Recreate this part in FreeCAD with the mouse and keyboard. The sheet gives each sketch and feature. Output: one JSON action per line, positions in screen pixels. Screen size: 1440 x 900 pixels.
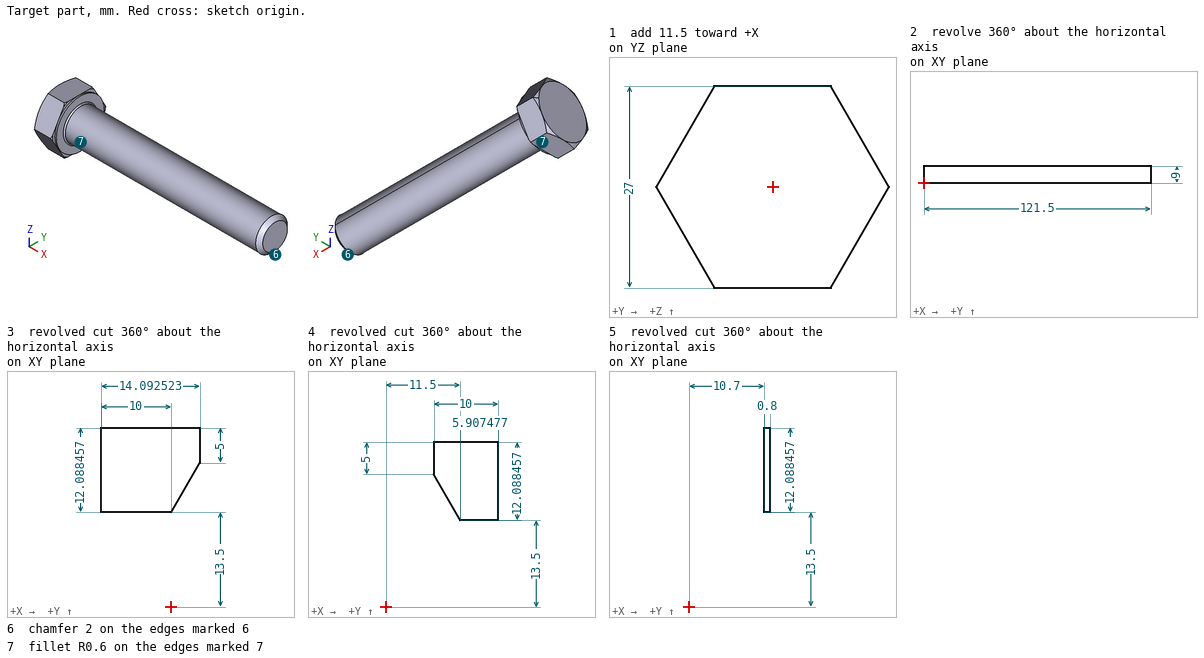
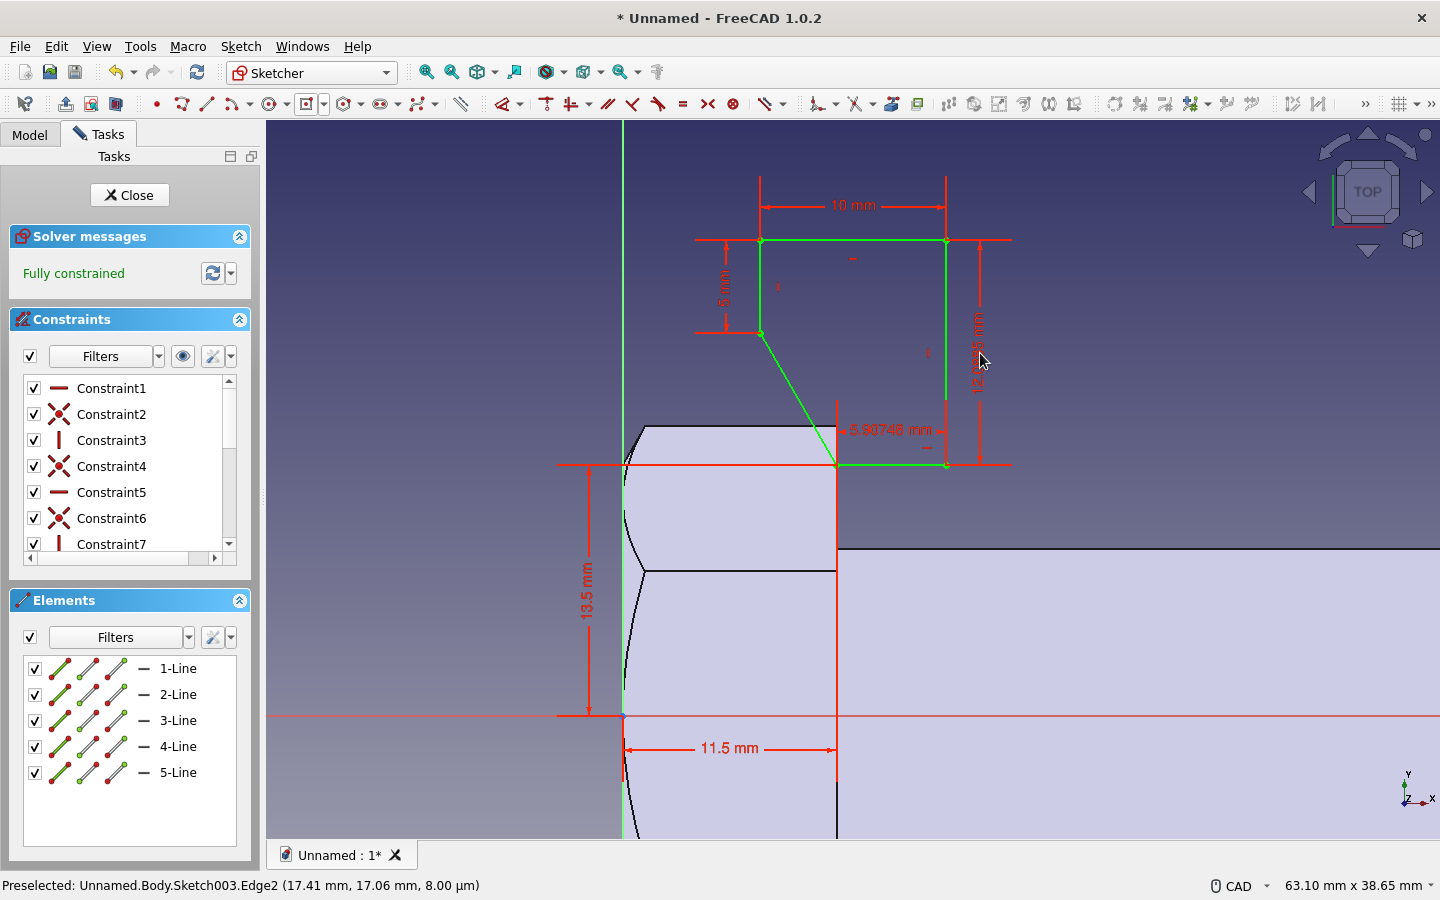
{"action": "left_click", "coordinate": [130, 195]}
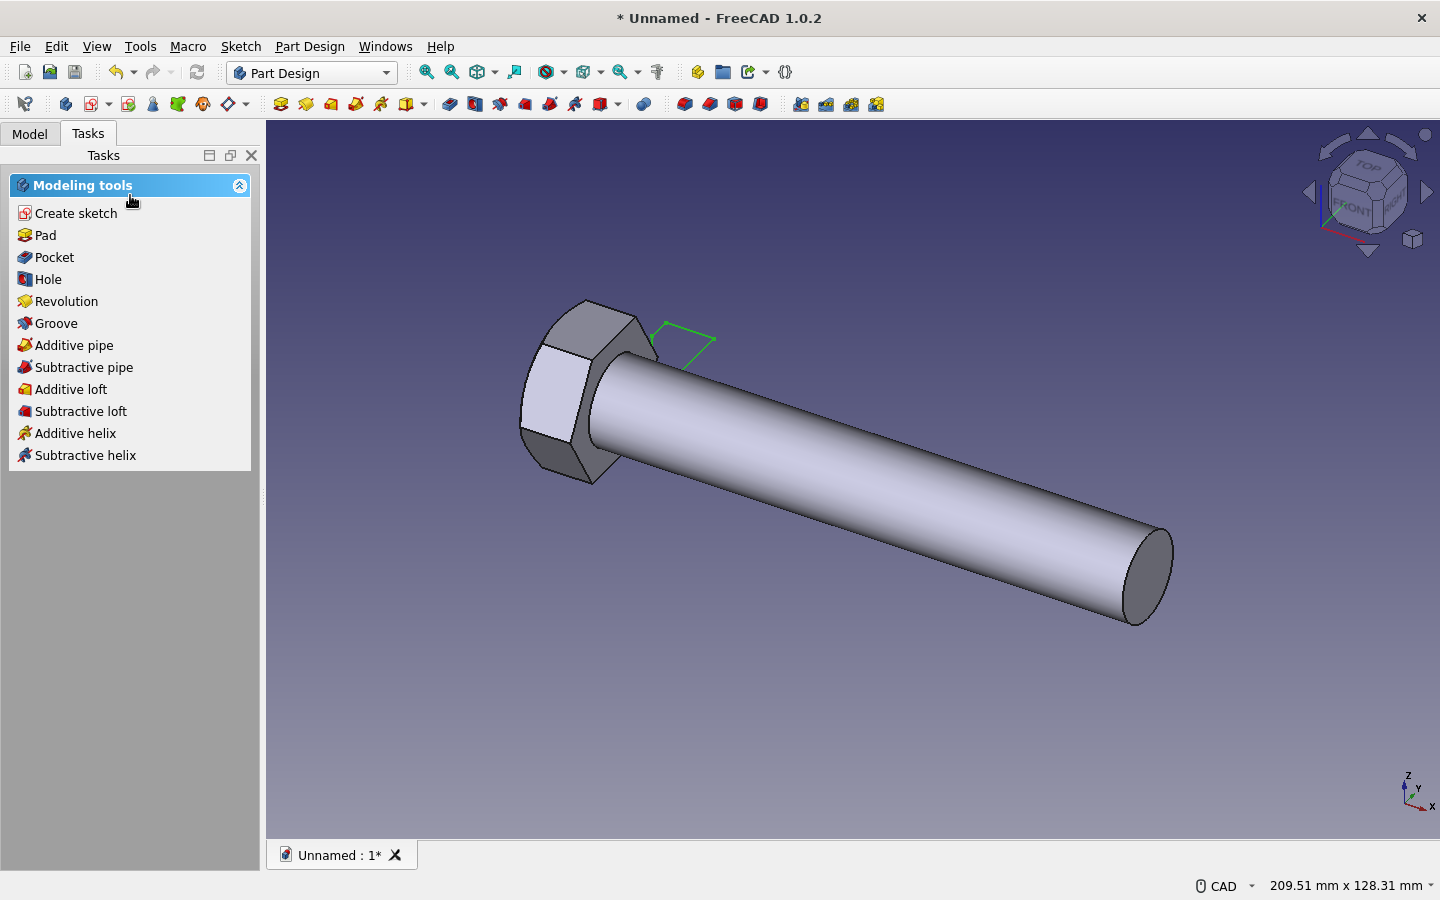
{"action": "left_click", "coordinate": [500, 104]}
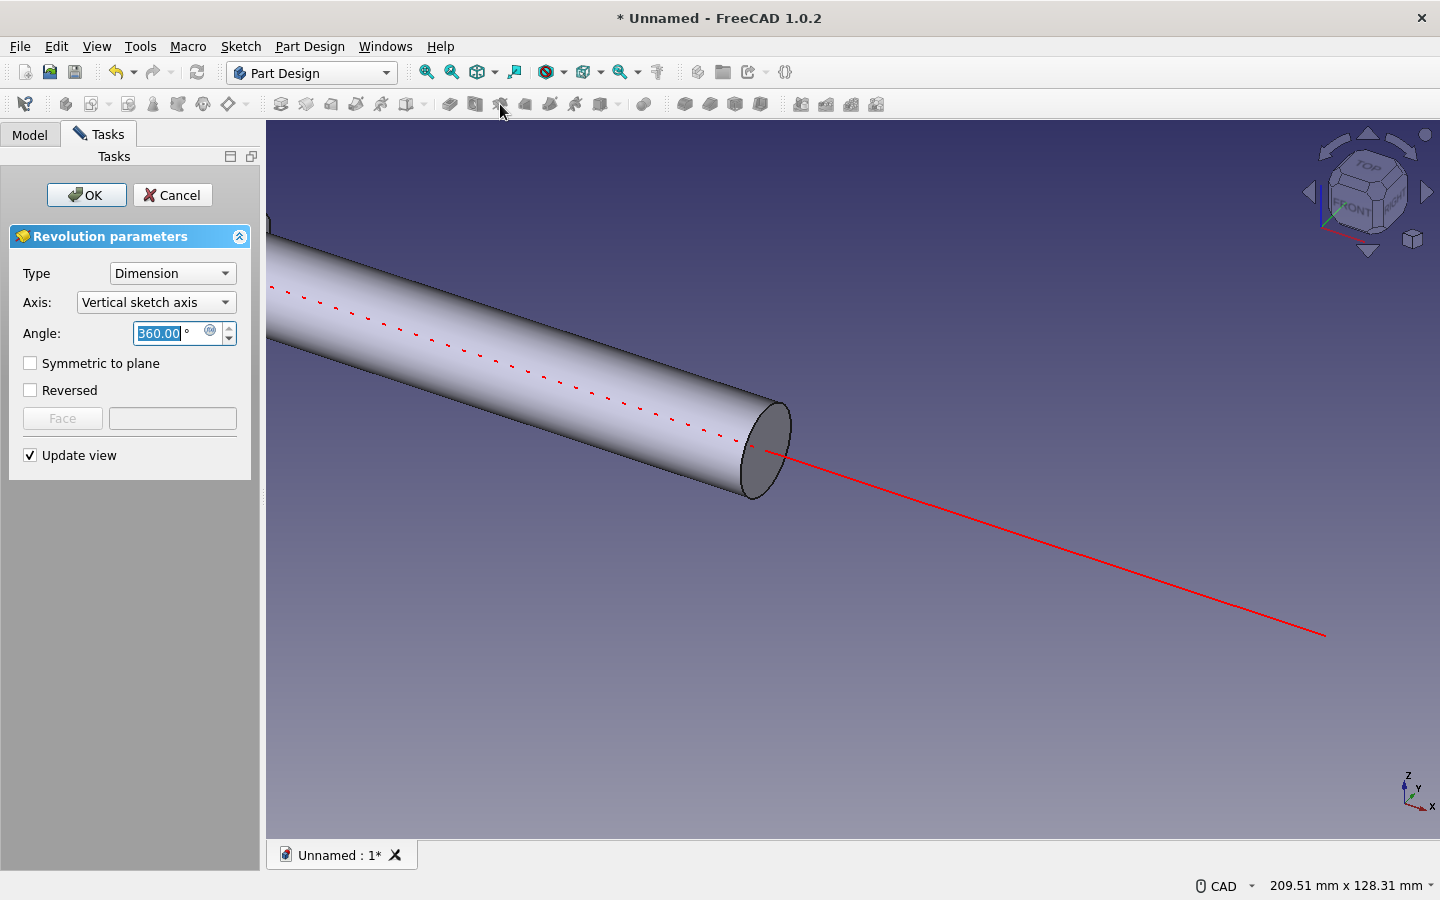
{"action": "left_click", "coordinate": [157, 302]}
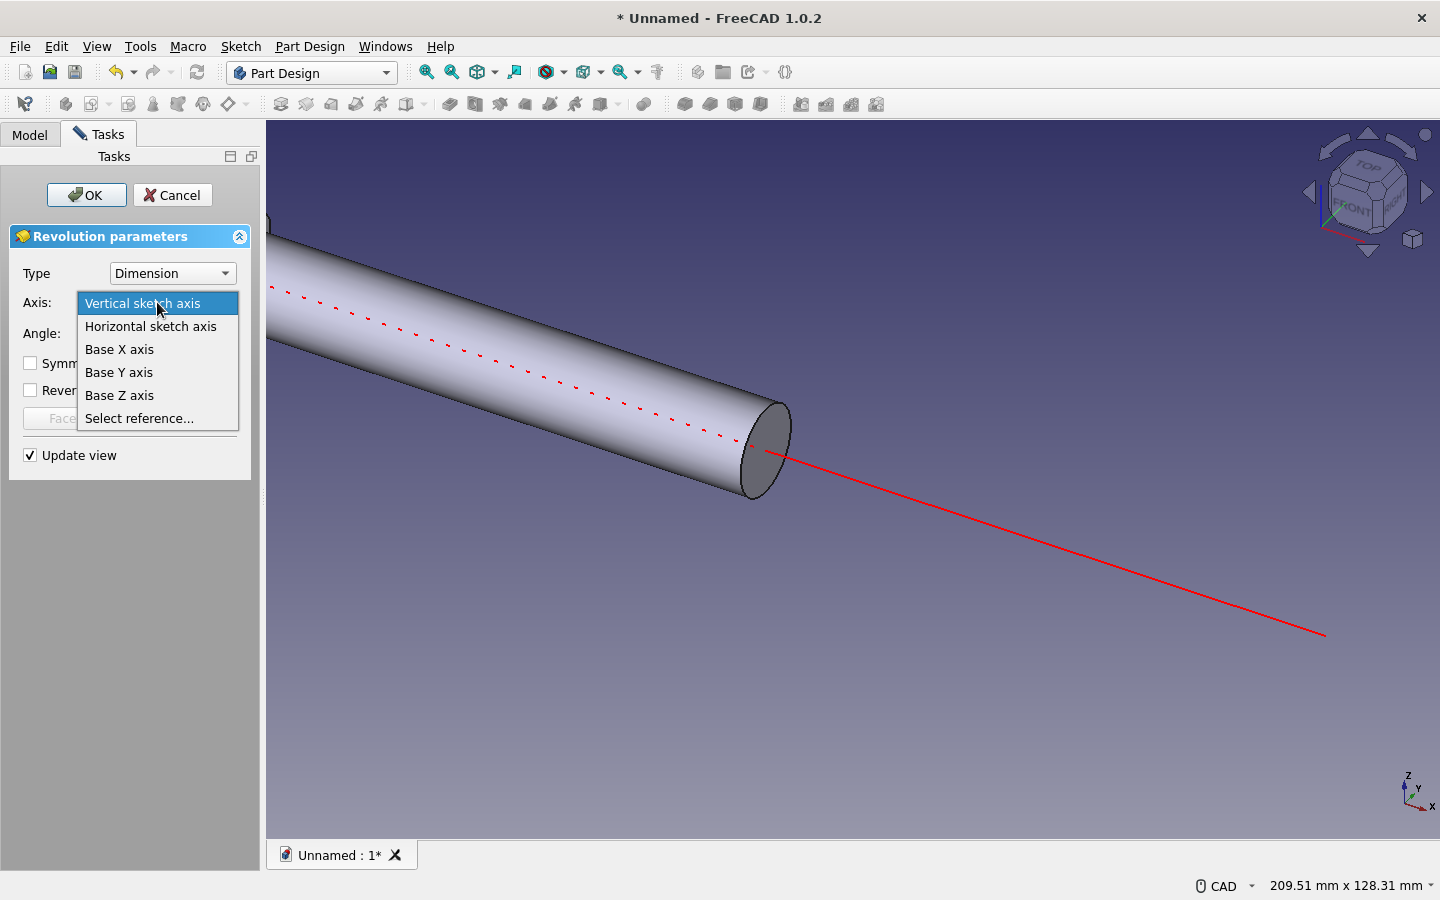
{"action": "left_click", "coordinate": [156, 326]}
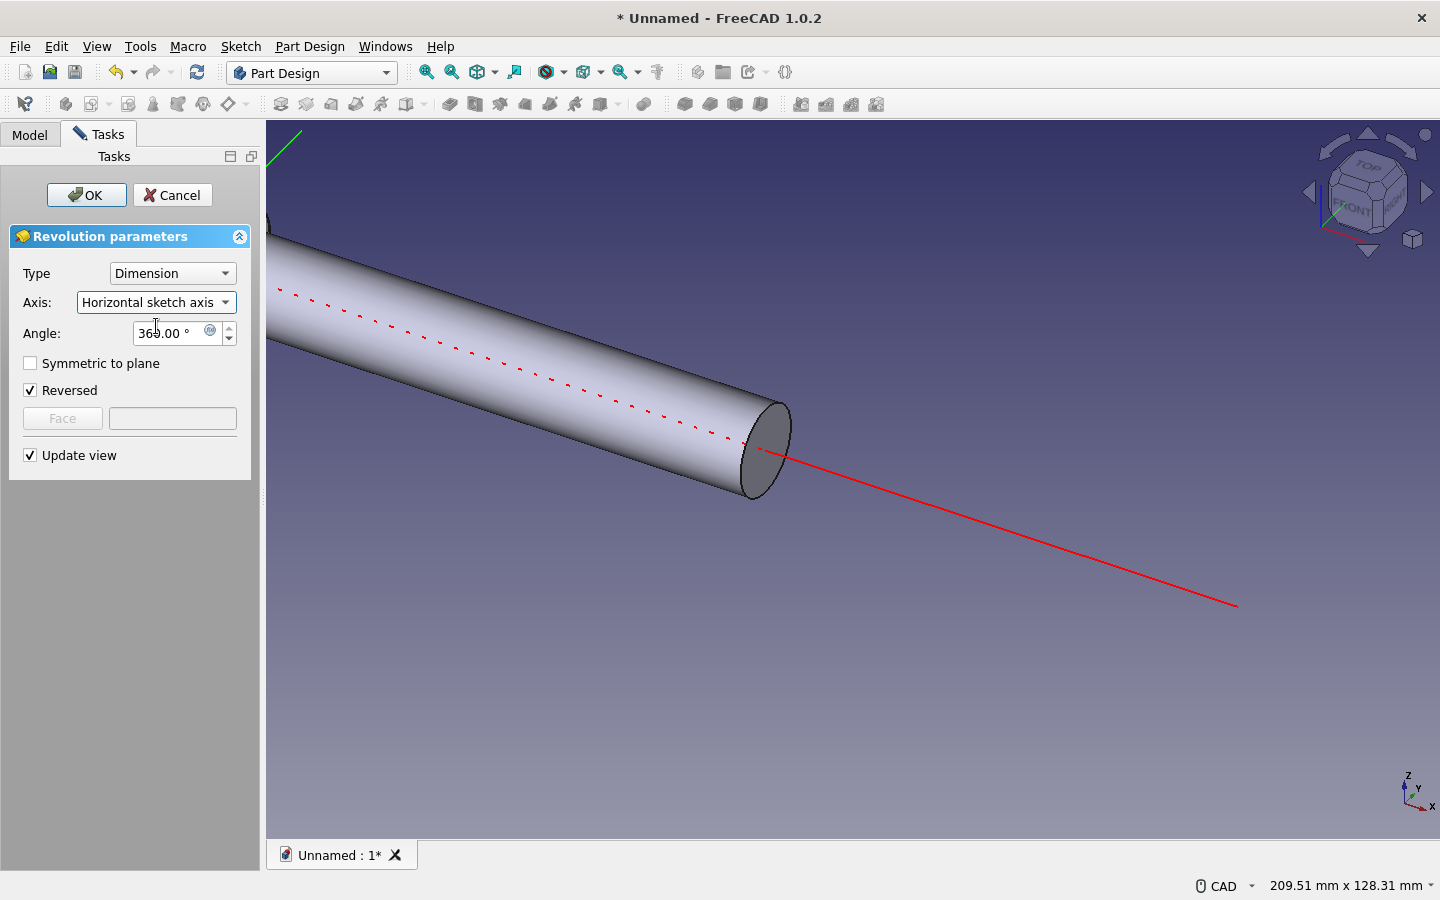
{"action": "left_click", "coordinate": [87, 195]}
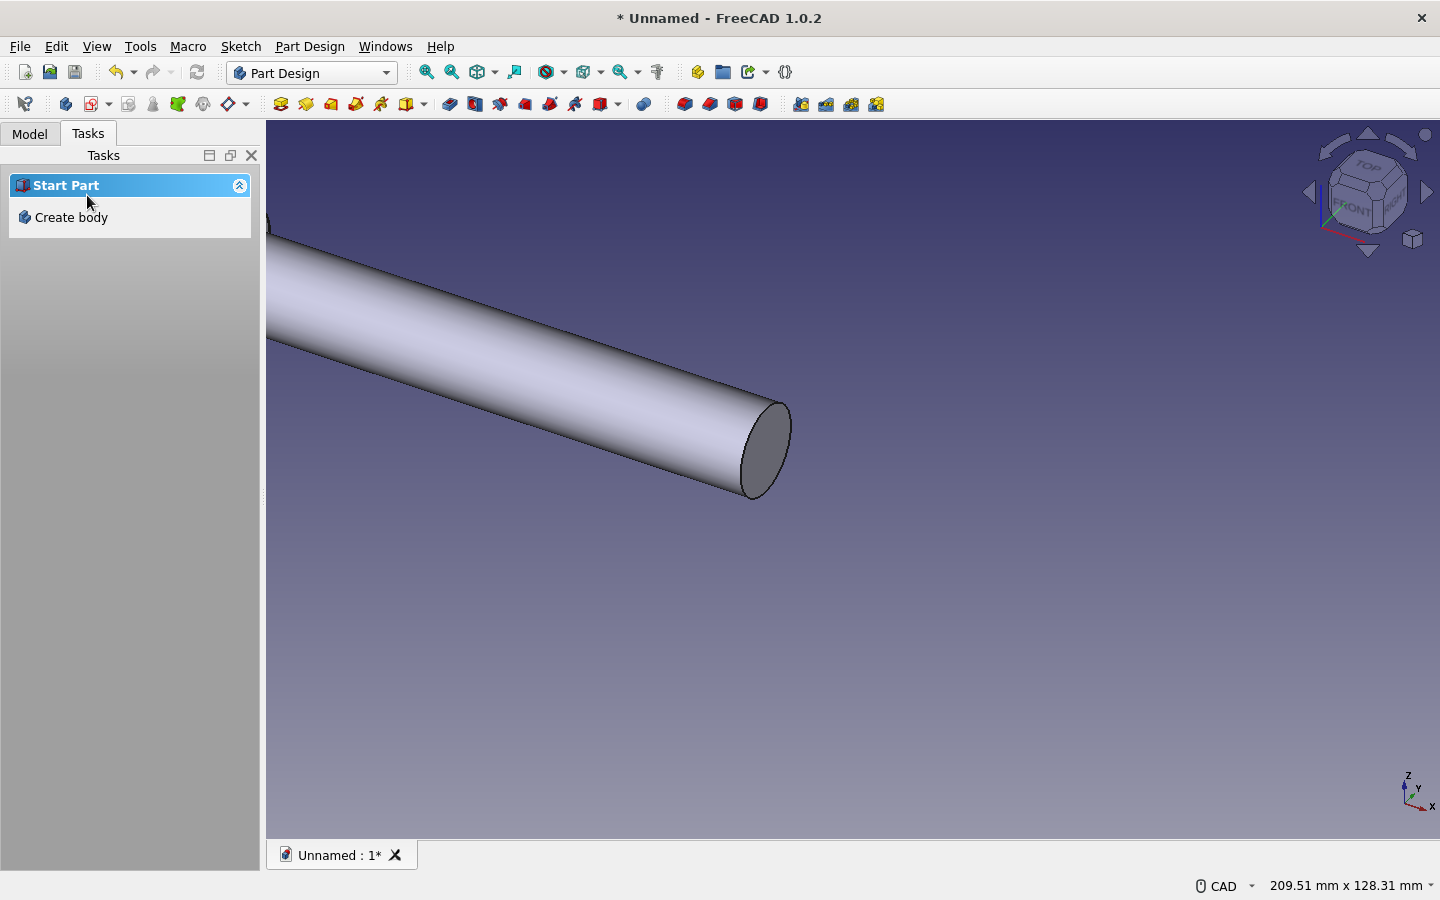
{"action": "left_click", "coordinate": [427, 72]}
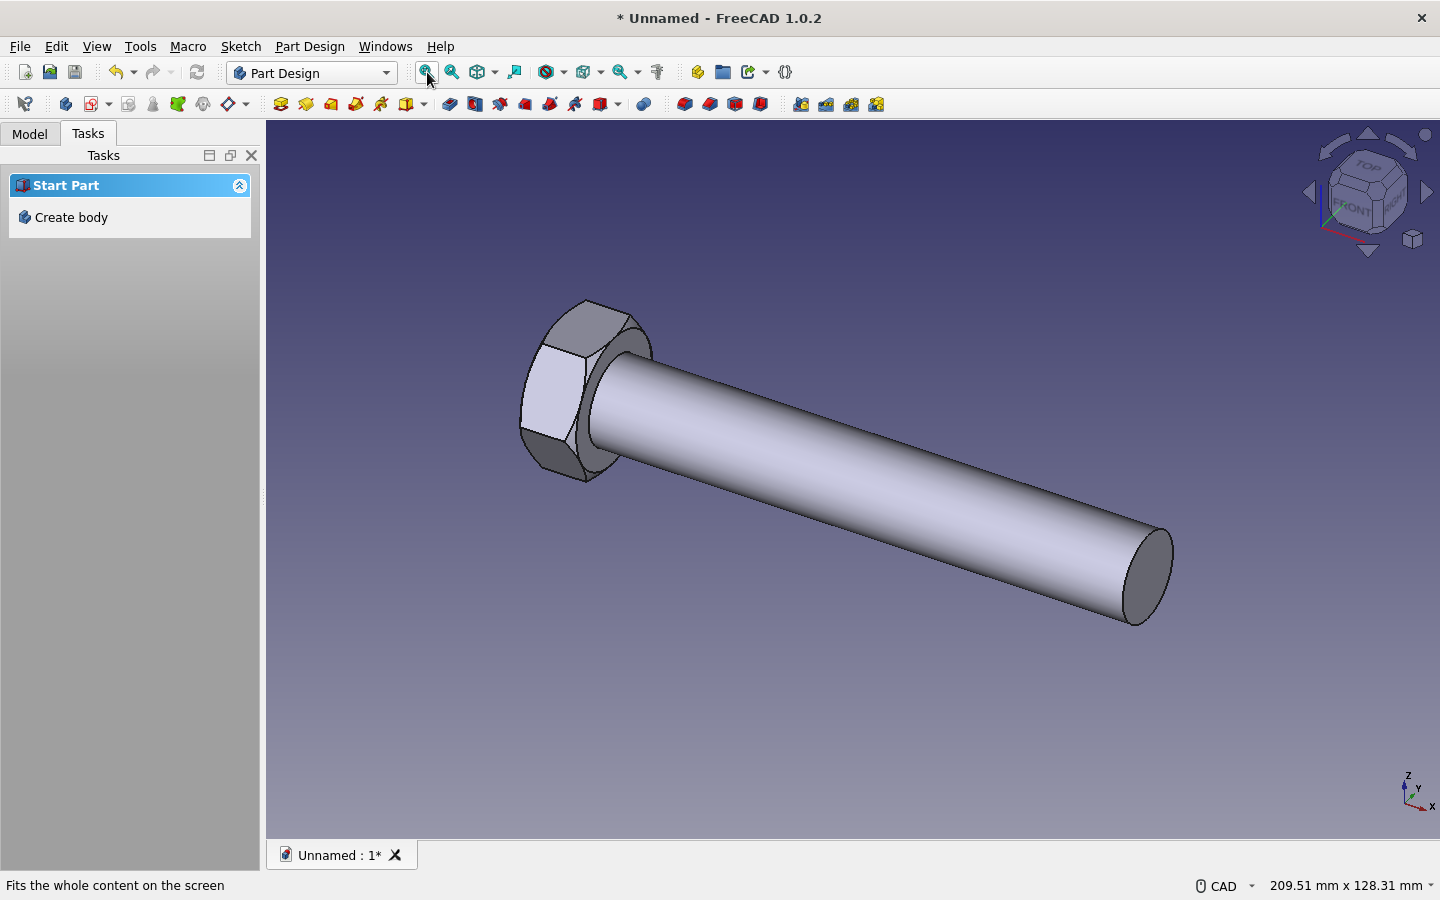
{"action": "left_click", "coordinate": [90, 104]}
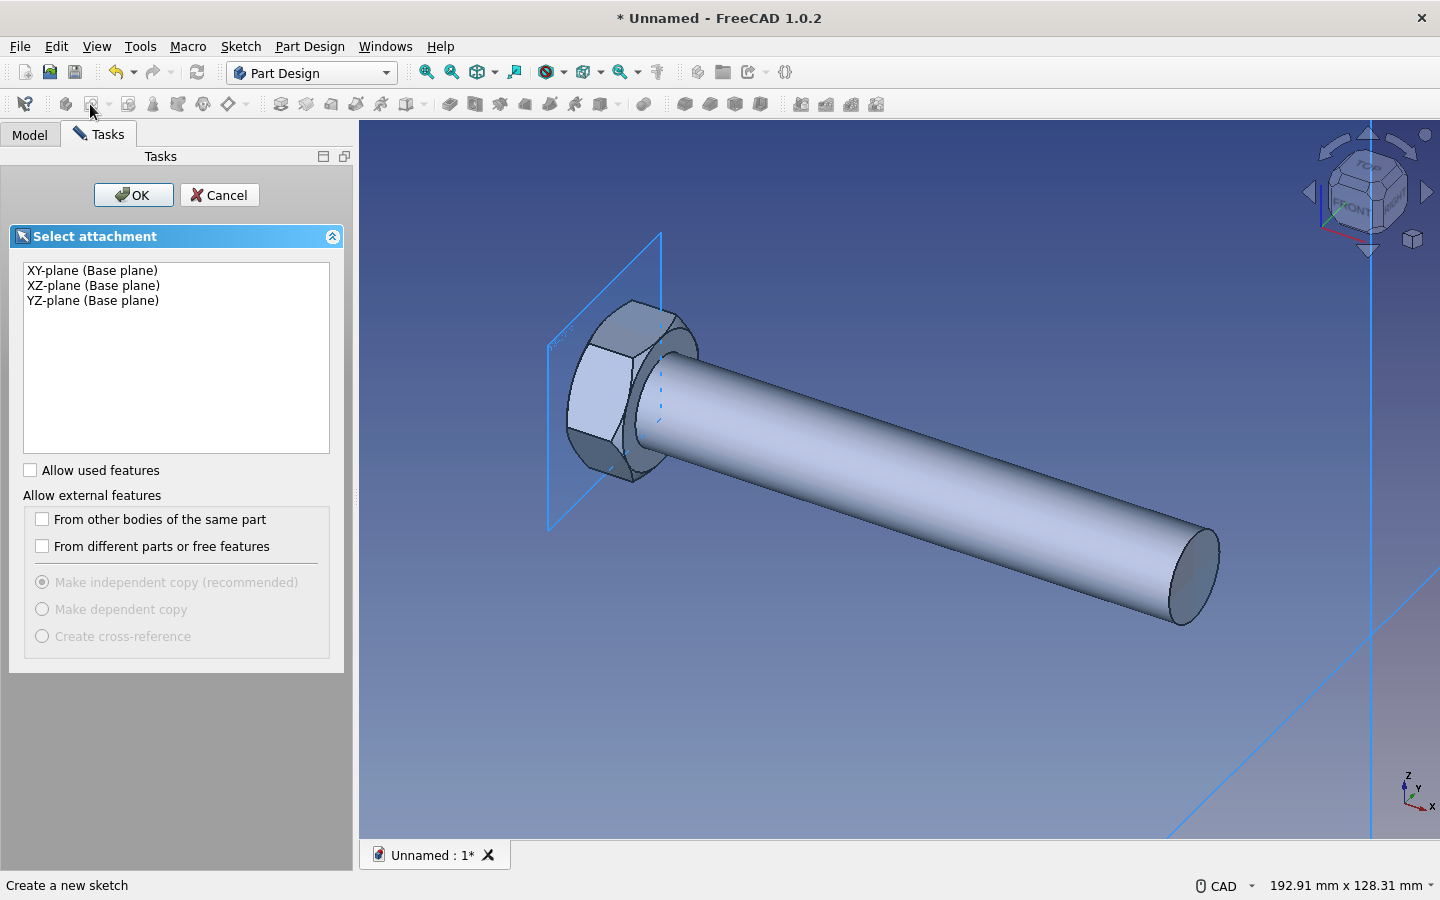
{"action": "left_click", "coordinate": [84, 270]}